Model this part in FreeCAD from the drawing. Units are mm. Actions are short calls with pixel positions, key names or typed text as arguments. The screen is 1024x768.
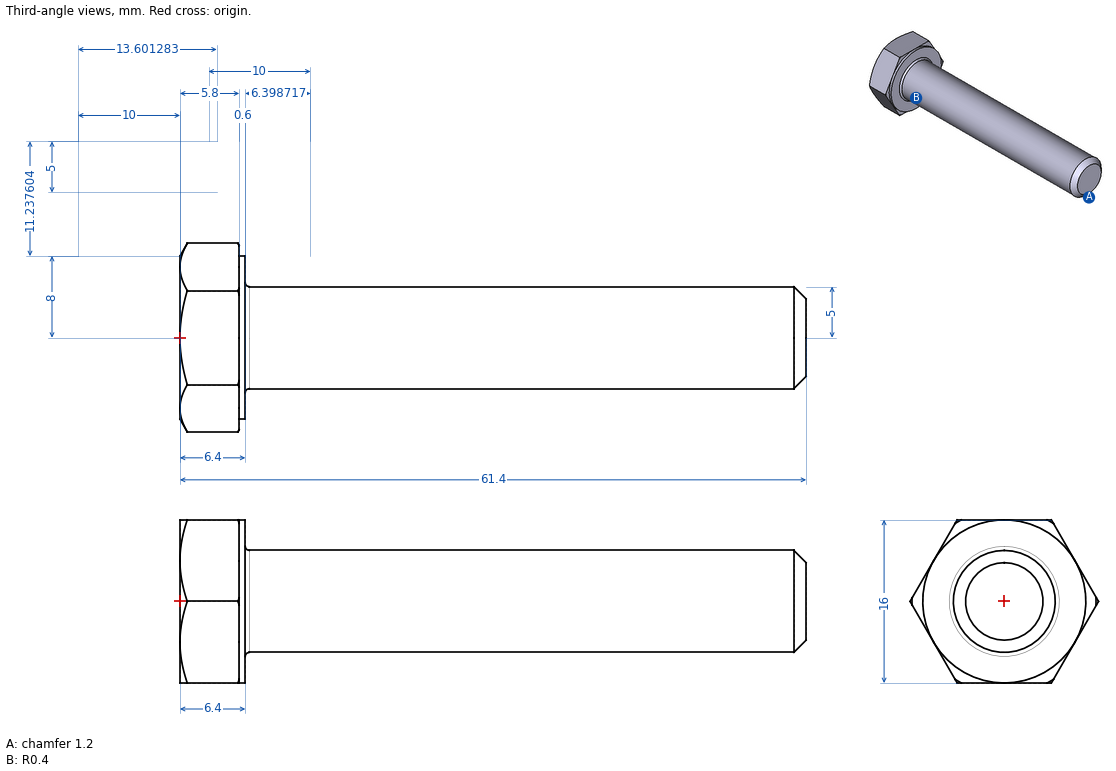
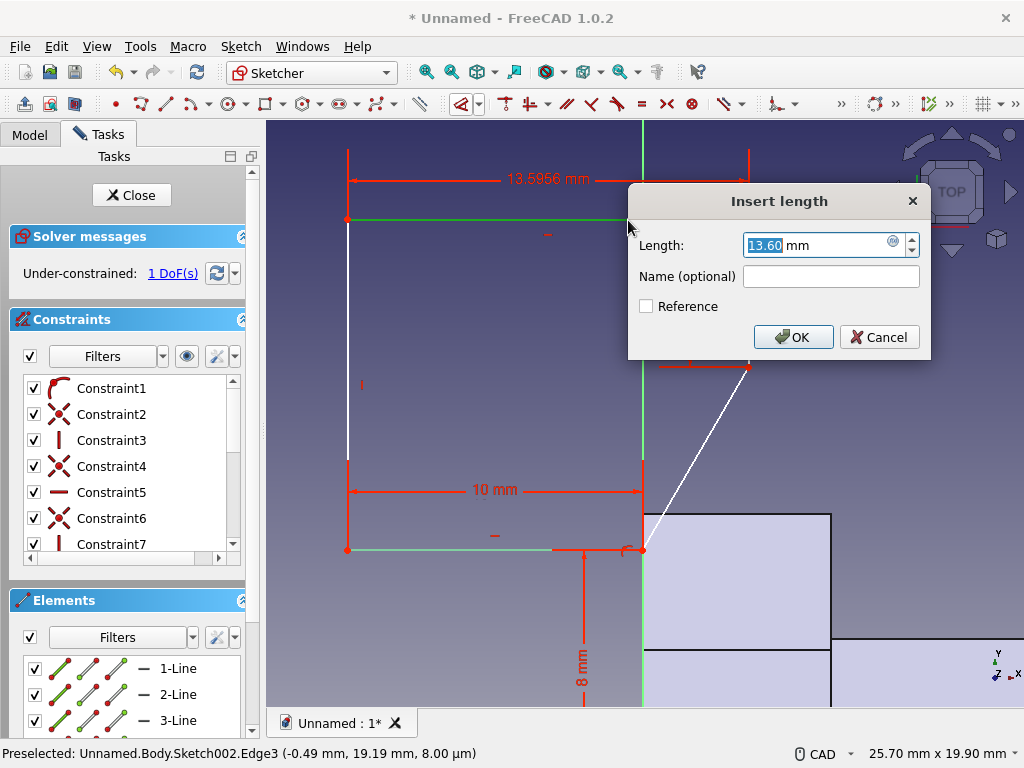
text(13.601283)
key(Return)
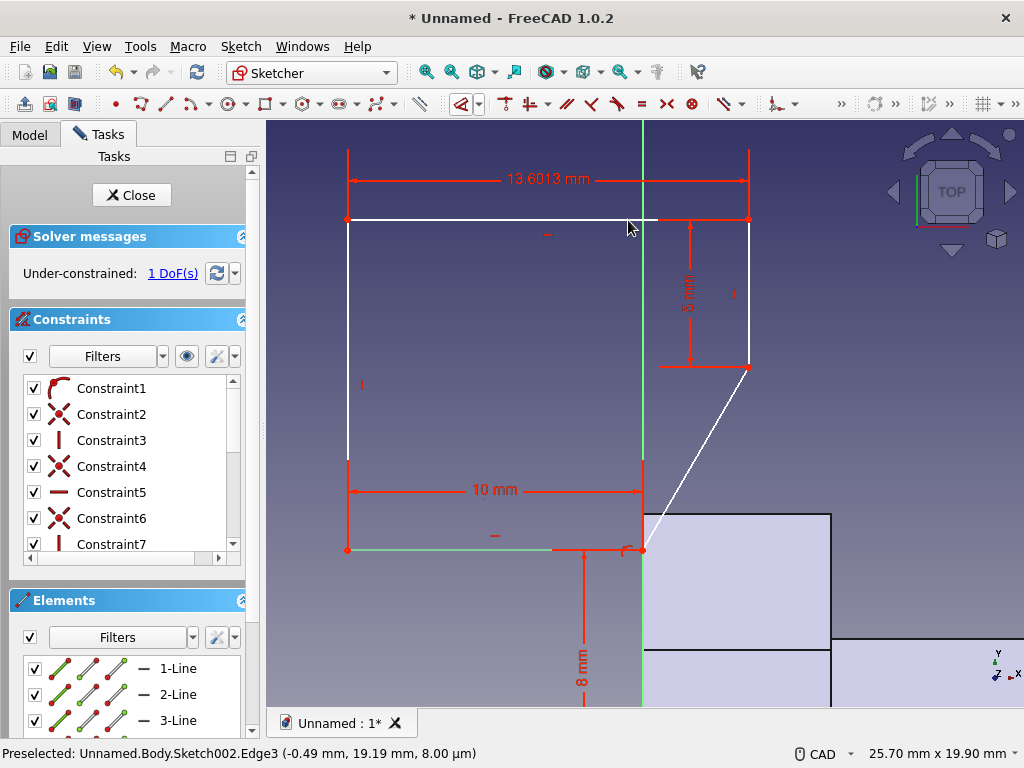
click(348, 319)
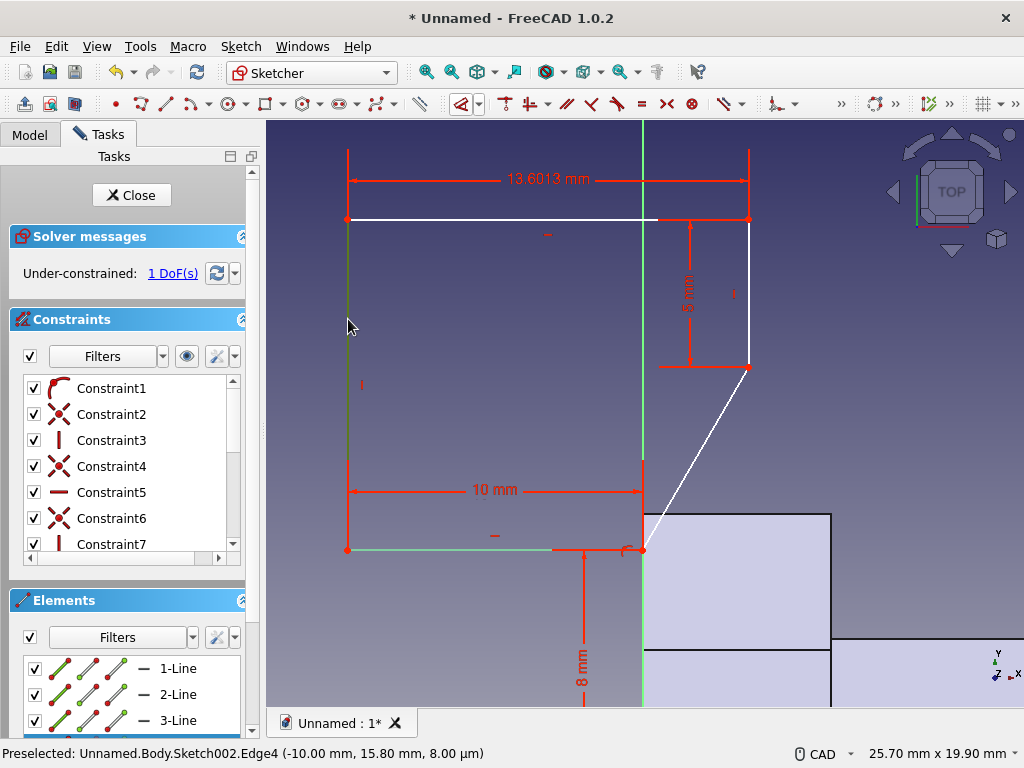
click(478, 104)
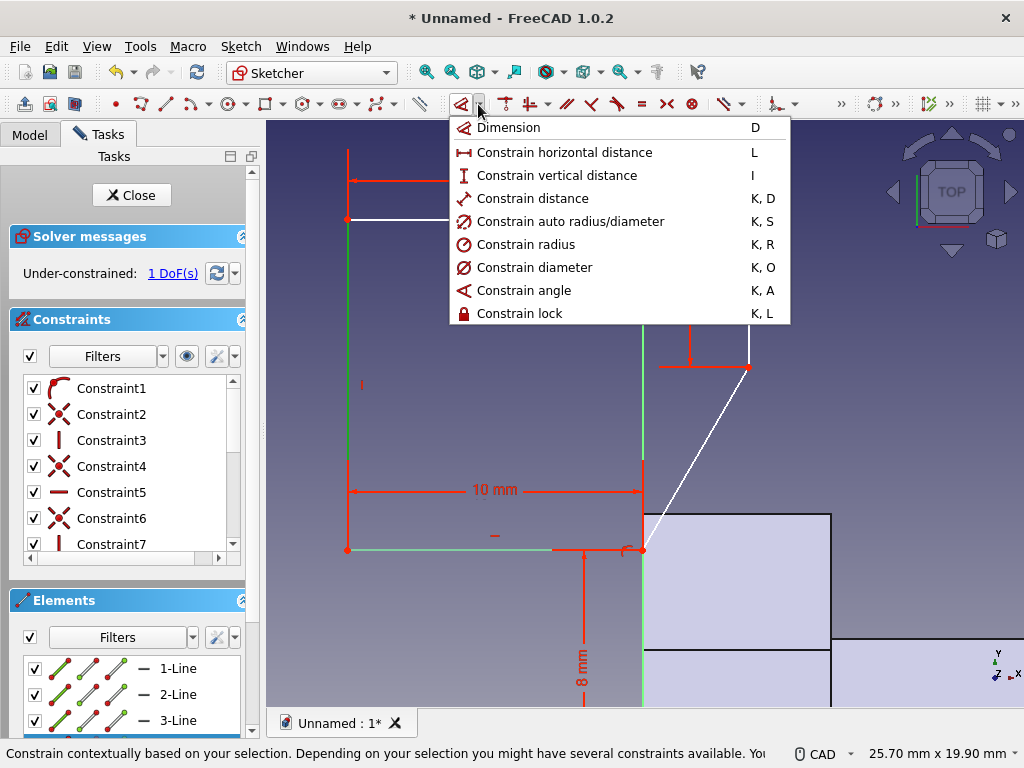
click(620, 176)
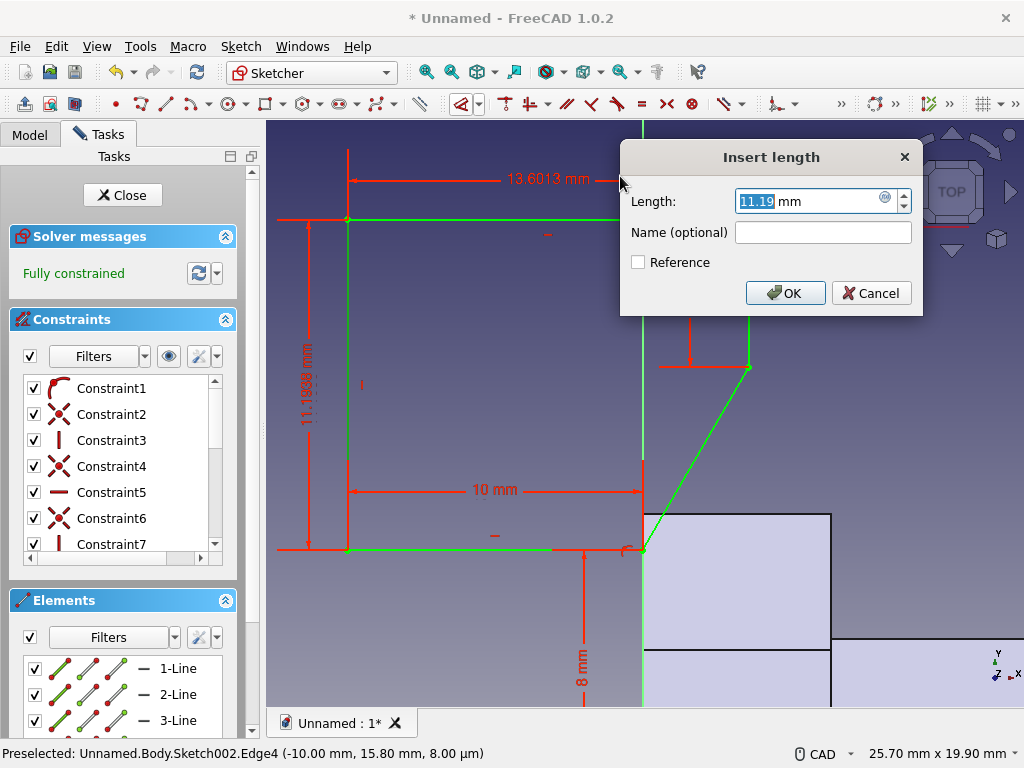
text(11.237604)
key(Return)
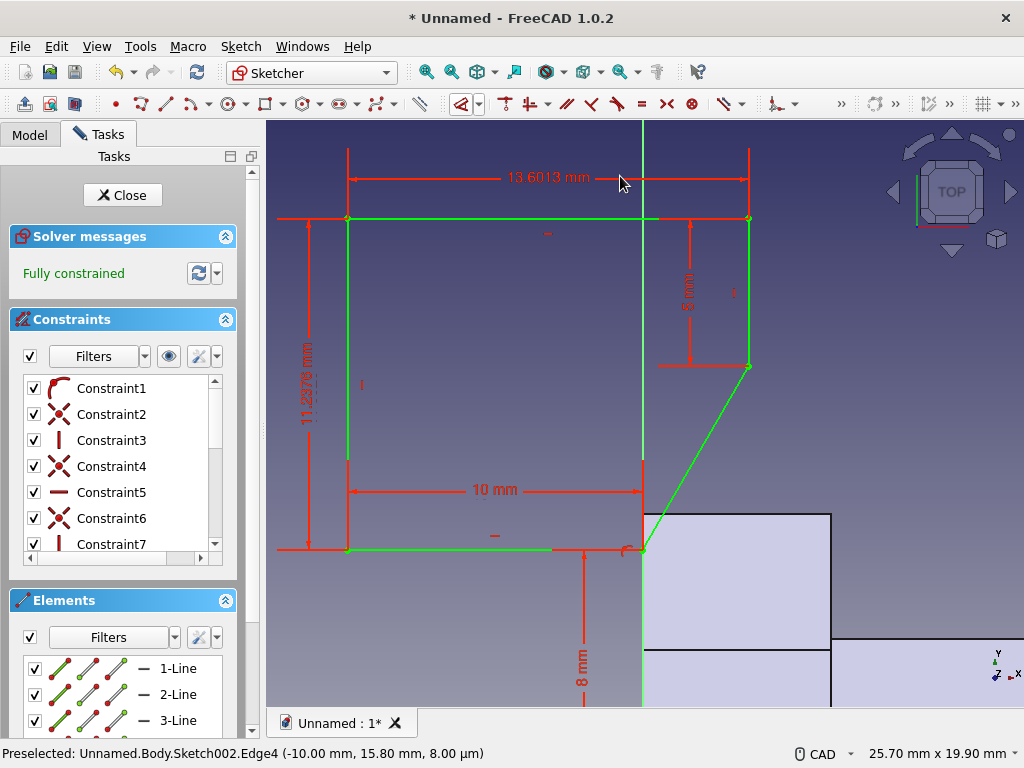
click(123, 195)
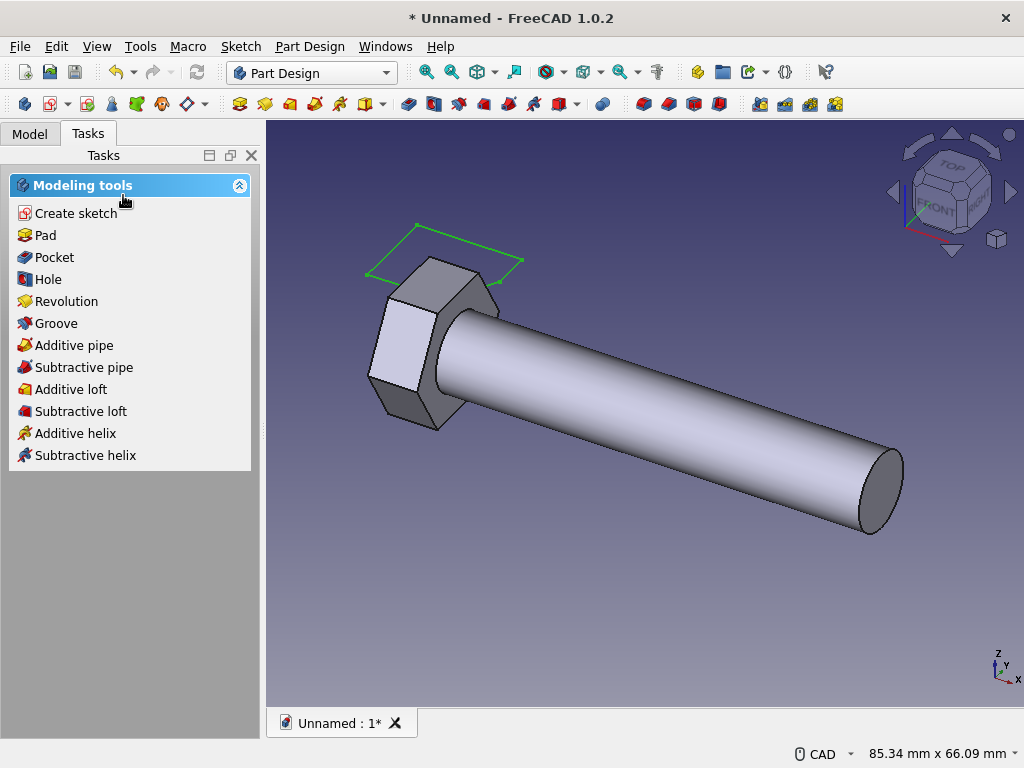
click(459, 104)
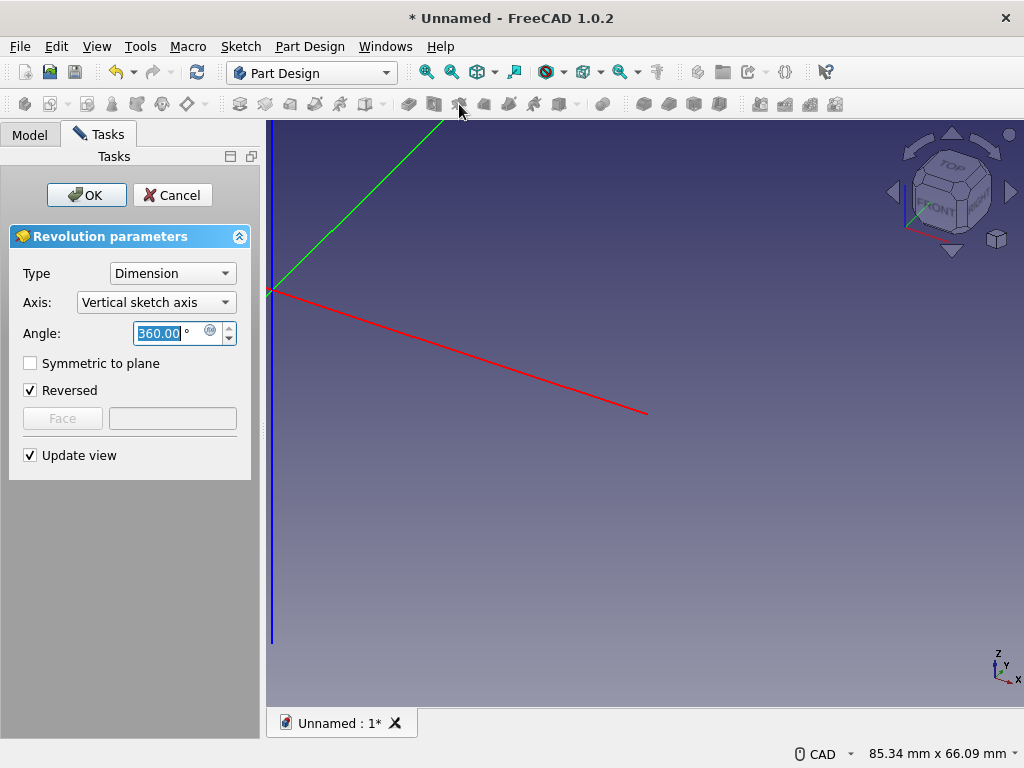
click(157, 302)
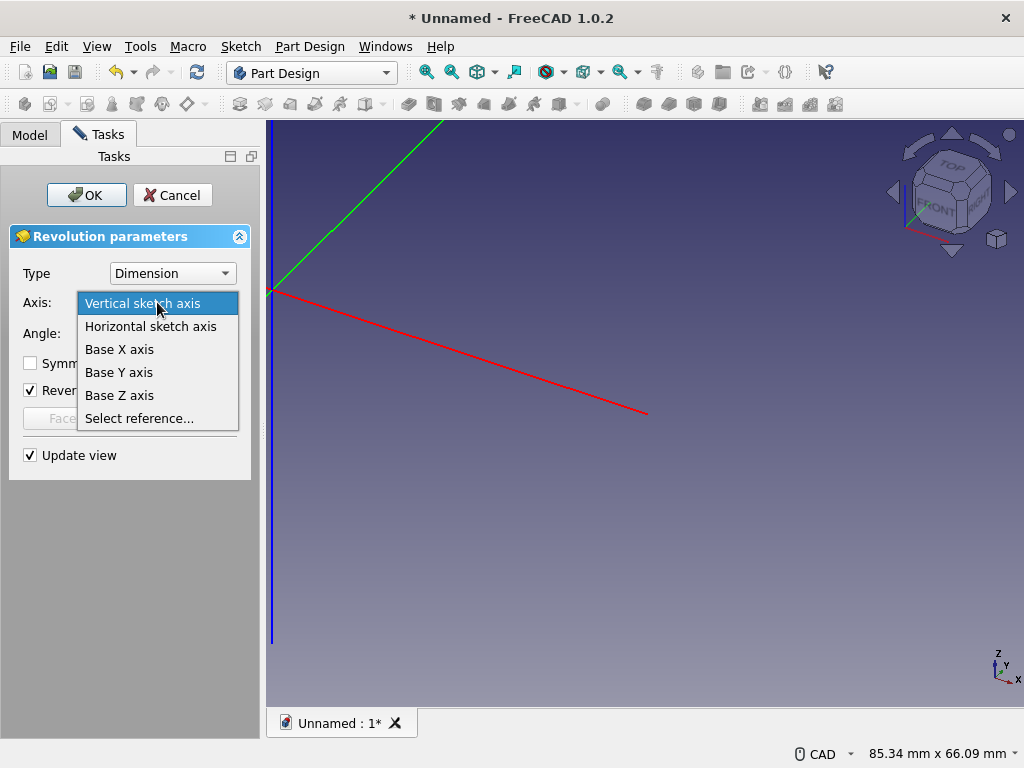
click(156, 326)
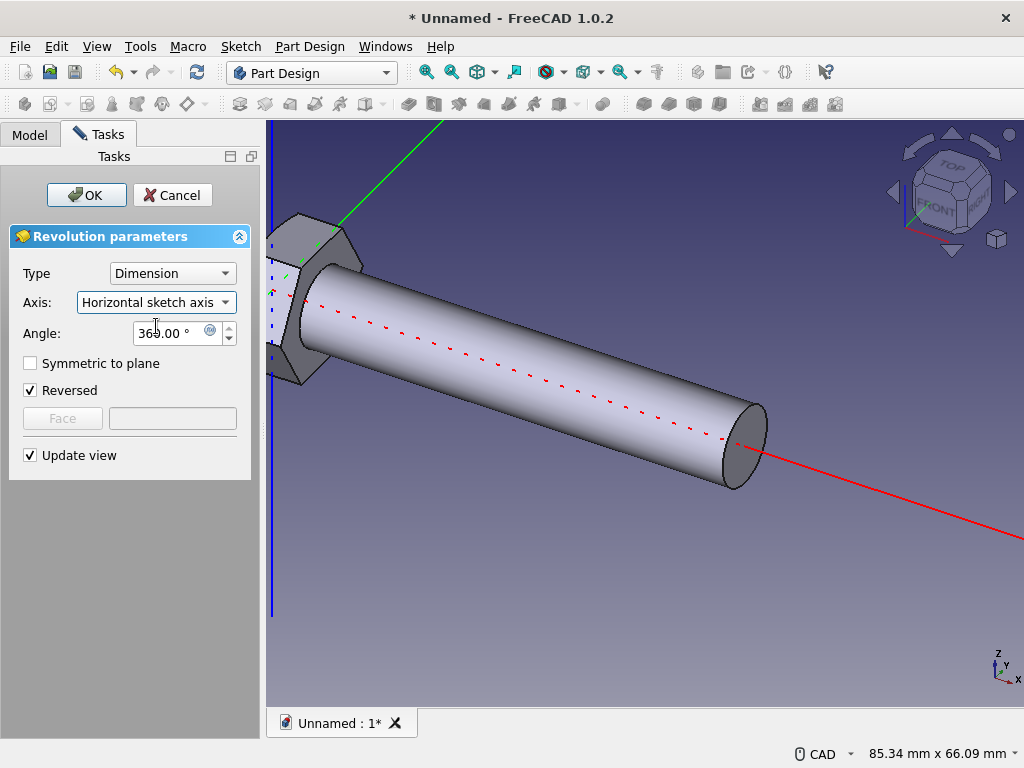
click(87, 195)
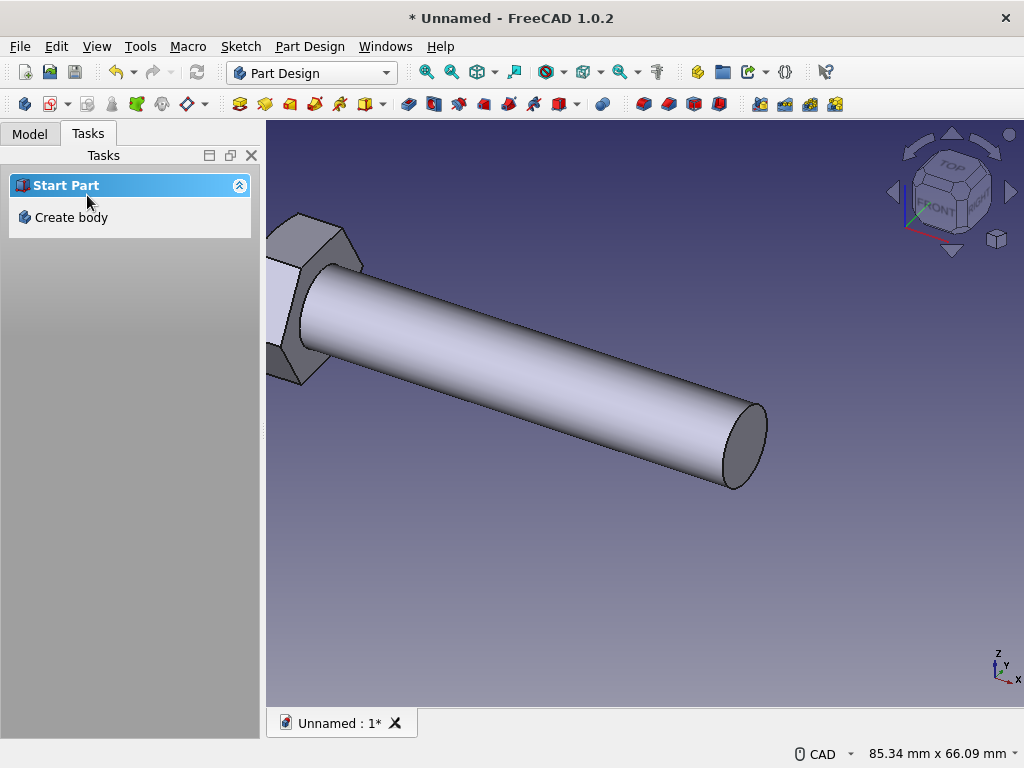
click(427, 72)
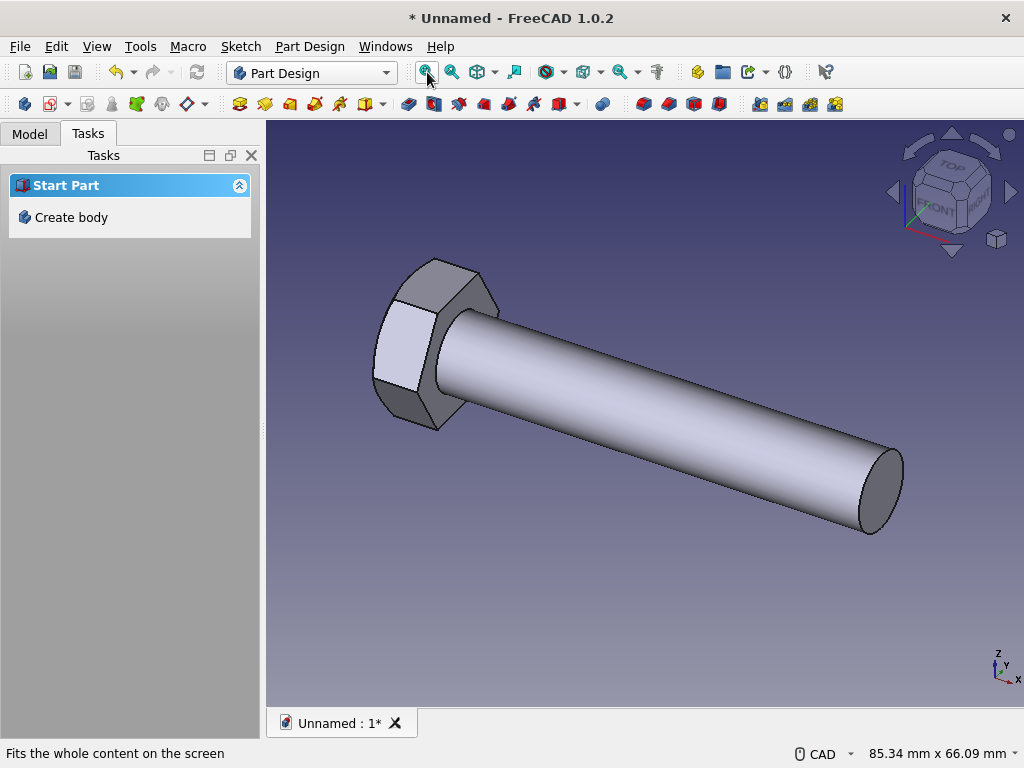
click(50, 104)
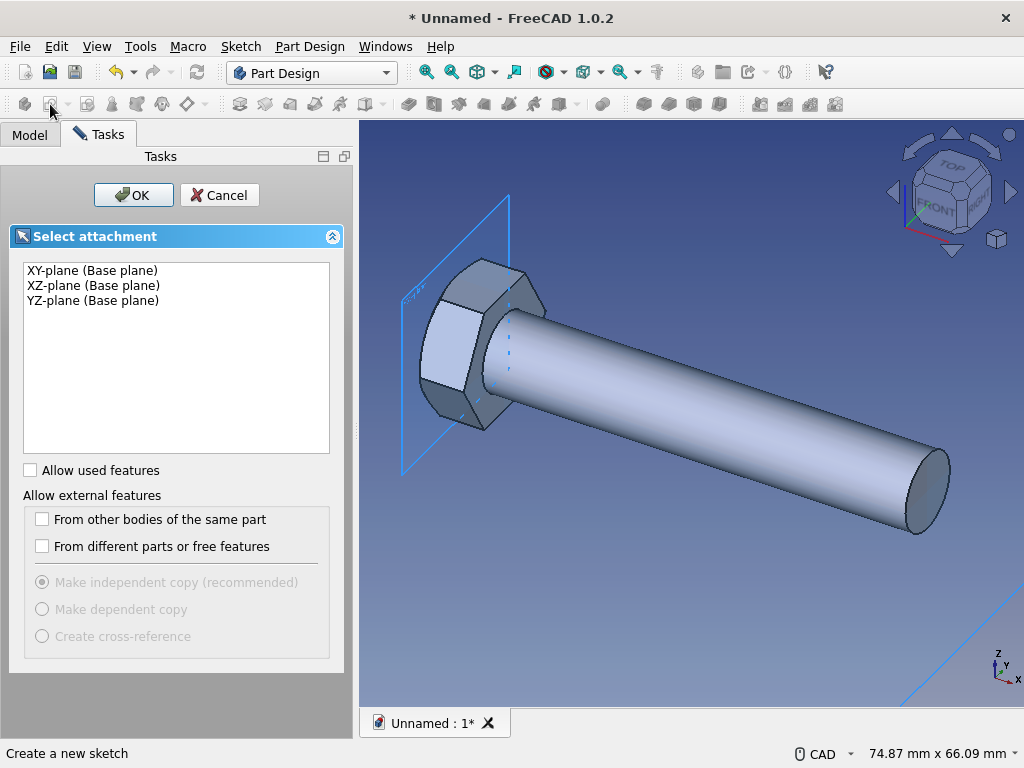
click(84, 270)